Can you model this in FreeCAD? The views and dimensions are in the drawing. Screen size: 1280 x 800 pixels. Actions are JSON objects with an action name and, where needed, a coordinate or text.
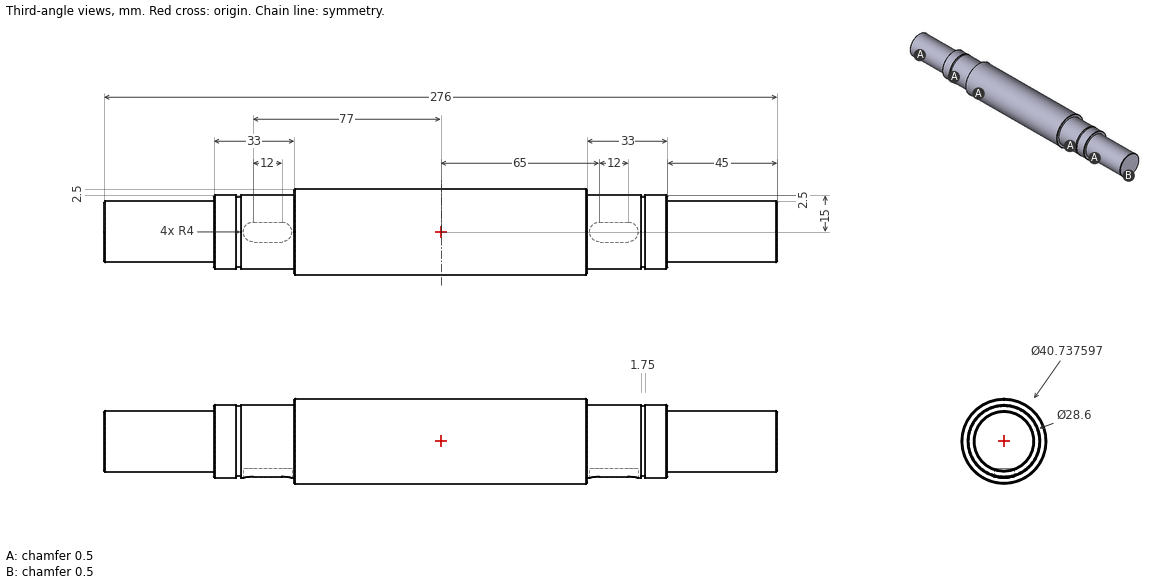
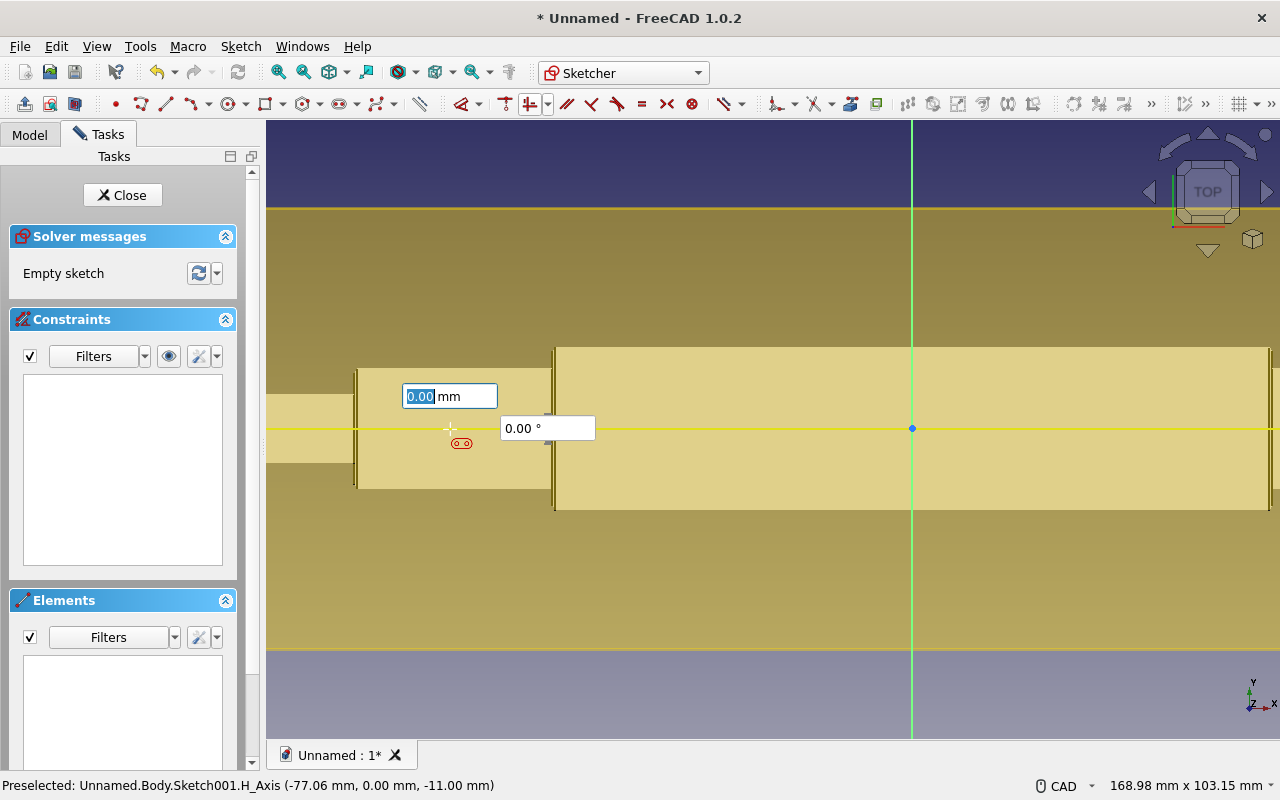
{"action": "left_click", "coordinate": [522, 420]}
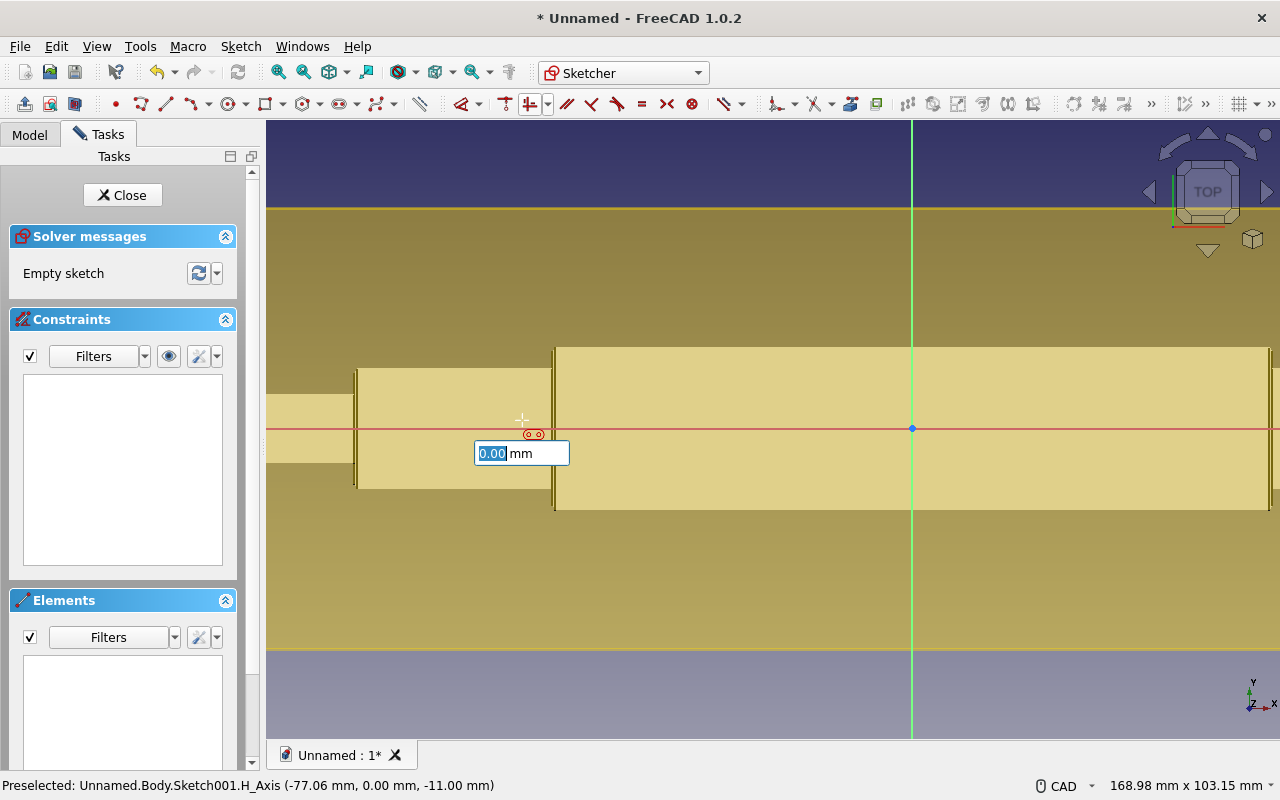
{"action": "left_click", "coordinate": [486, 405]}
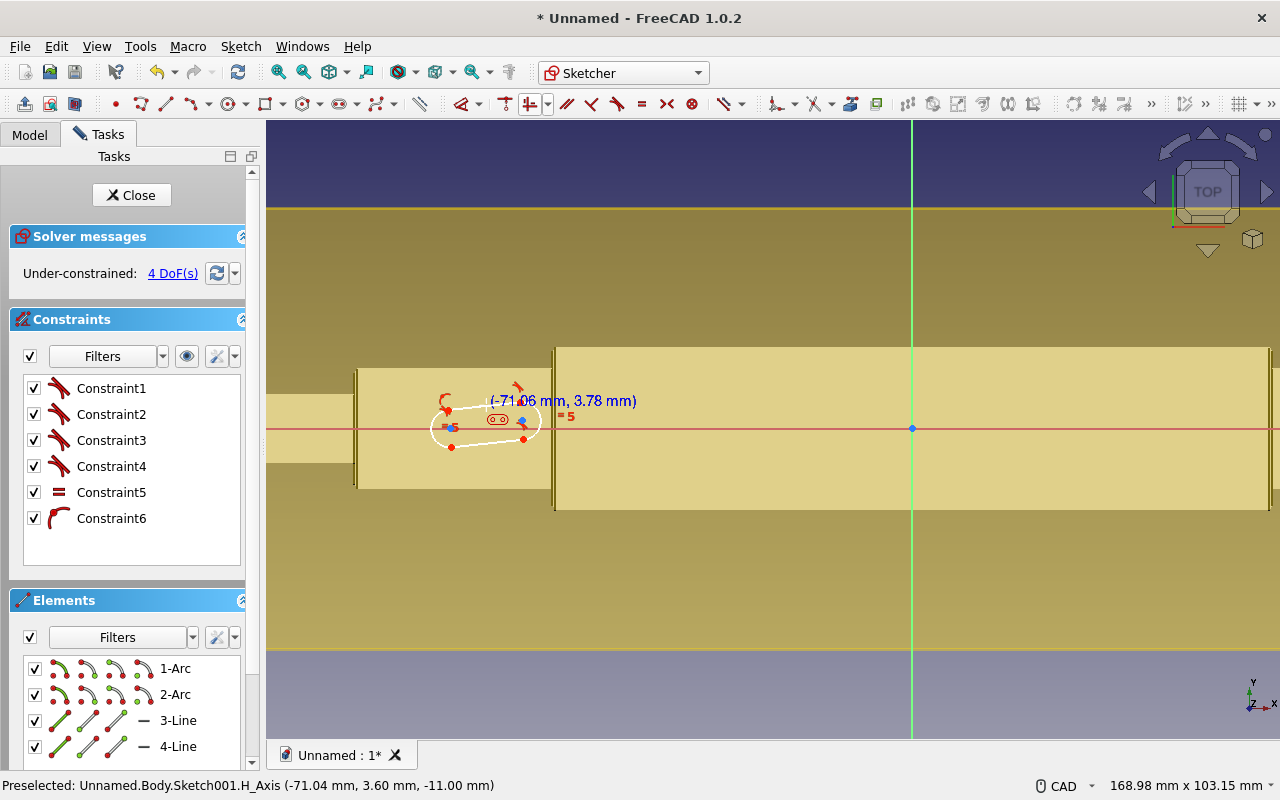
{"action": "scroll", "coordinate": [452, 431], "scroll_direction": "down", "scroll_amount": 3}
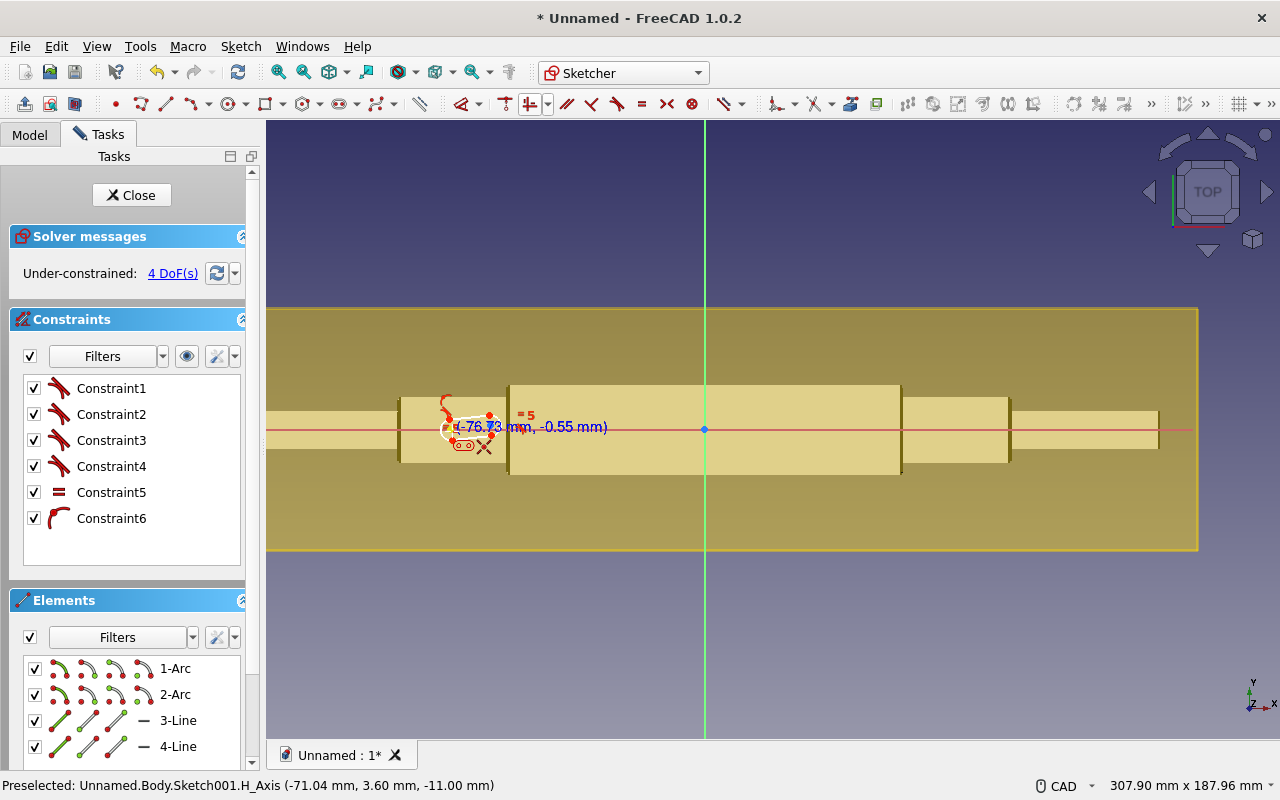
{"action": "scroll", "coordinate": [919, 430], "scroll_direction": "up", "scroll_amount": 3}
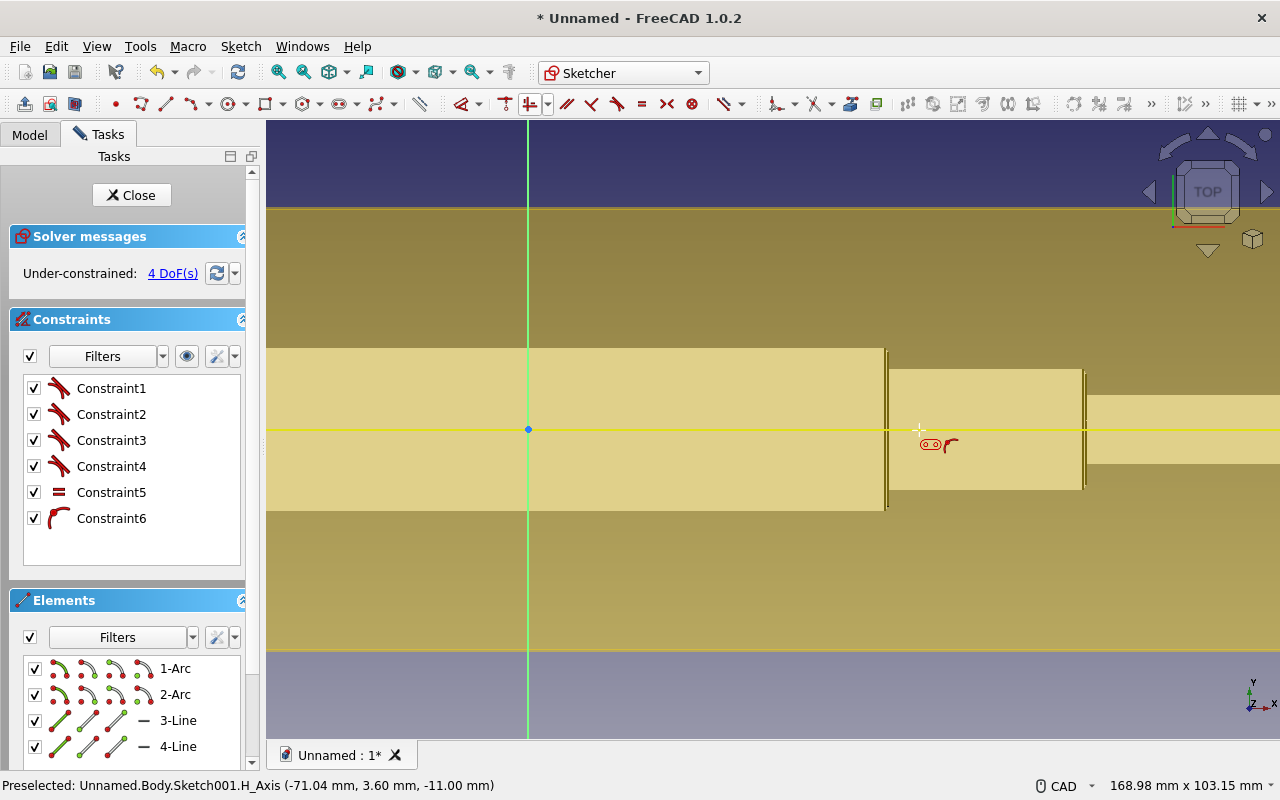
{"action": "left_click", "coordinate": [918, 430]}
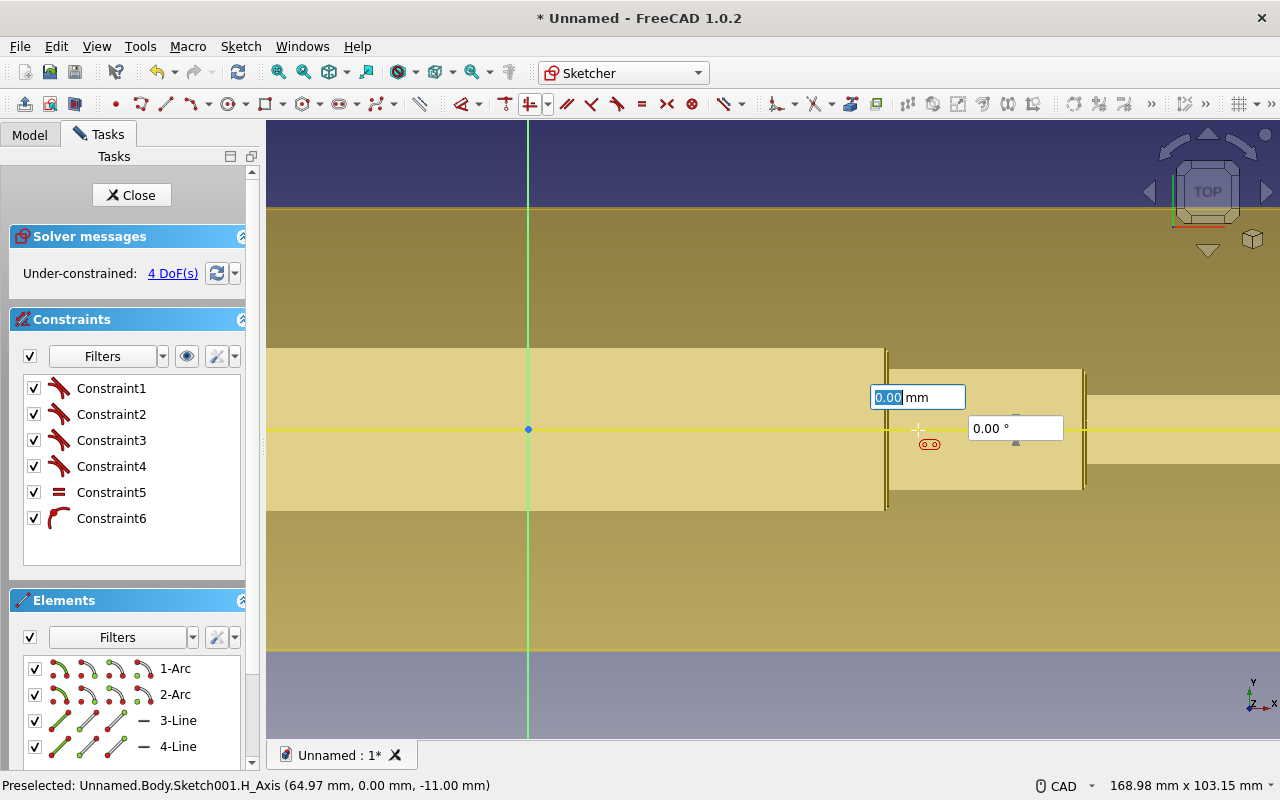
{"action": "left_click", "coordinate": [990, 421]}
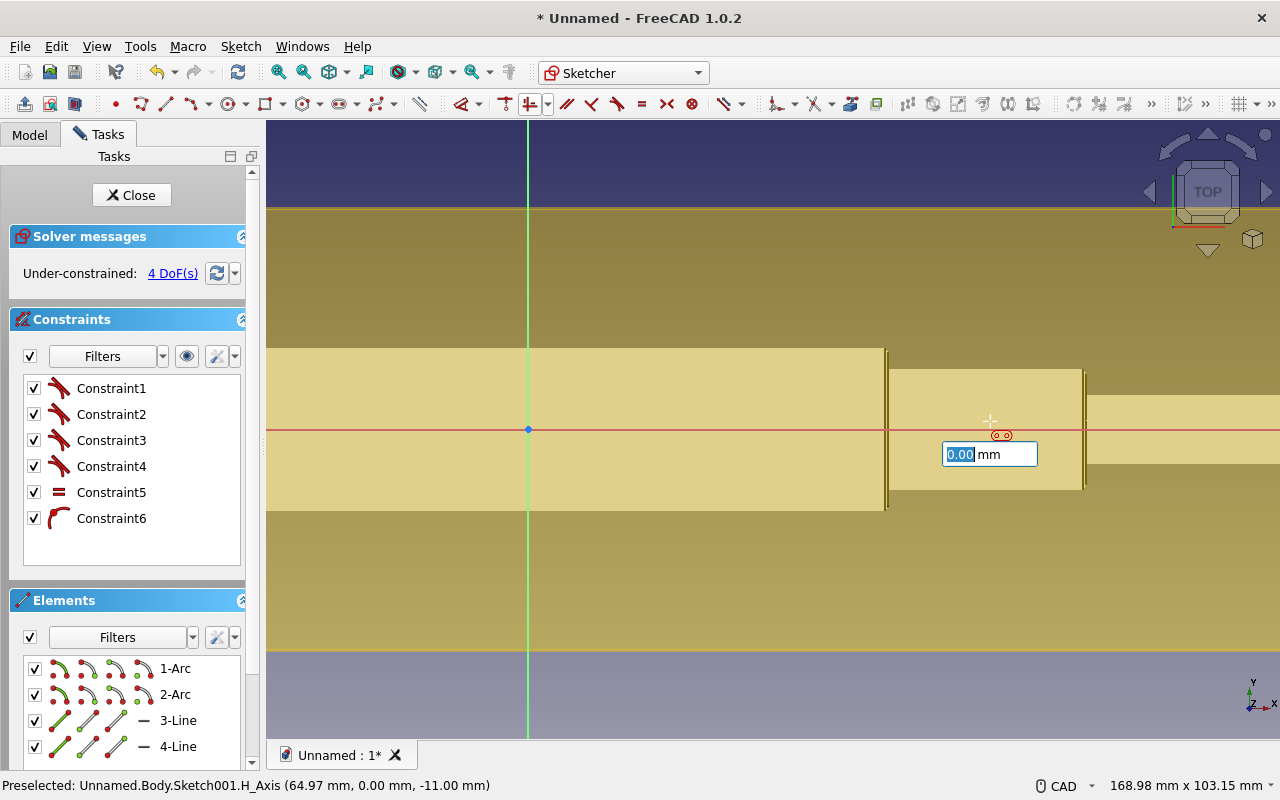
{"action": "left_click", "coordinate": [954, 405]}
{"action": "key", "text": "Escape"}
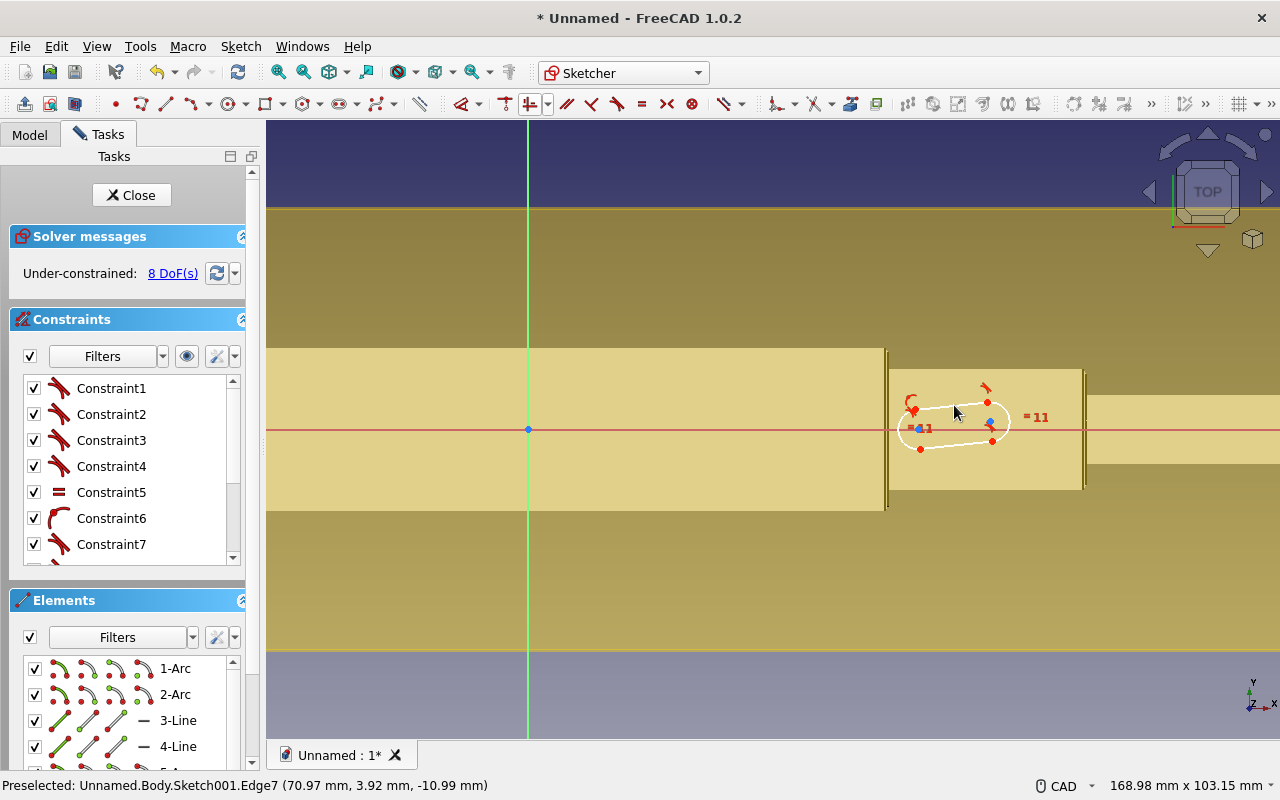
{"action": "scroll", "coordinate": [919, 429], "scroll_direction": "down", "scroll_amount": 3}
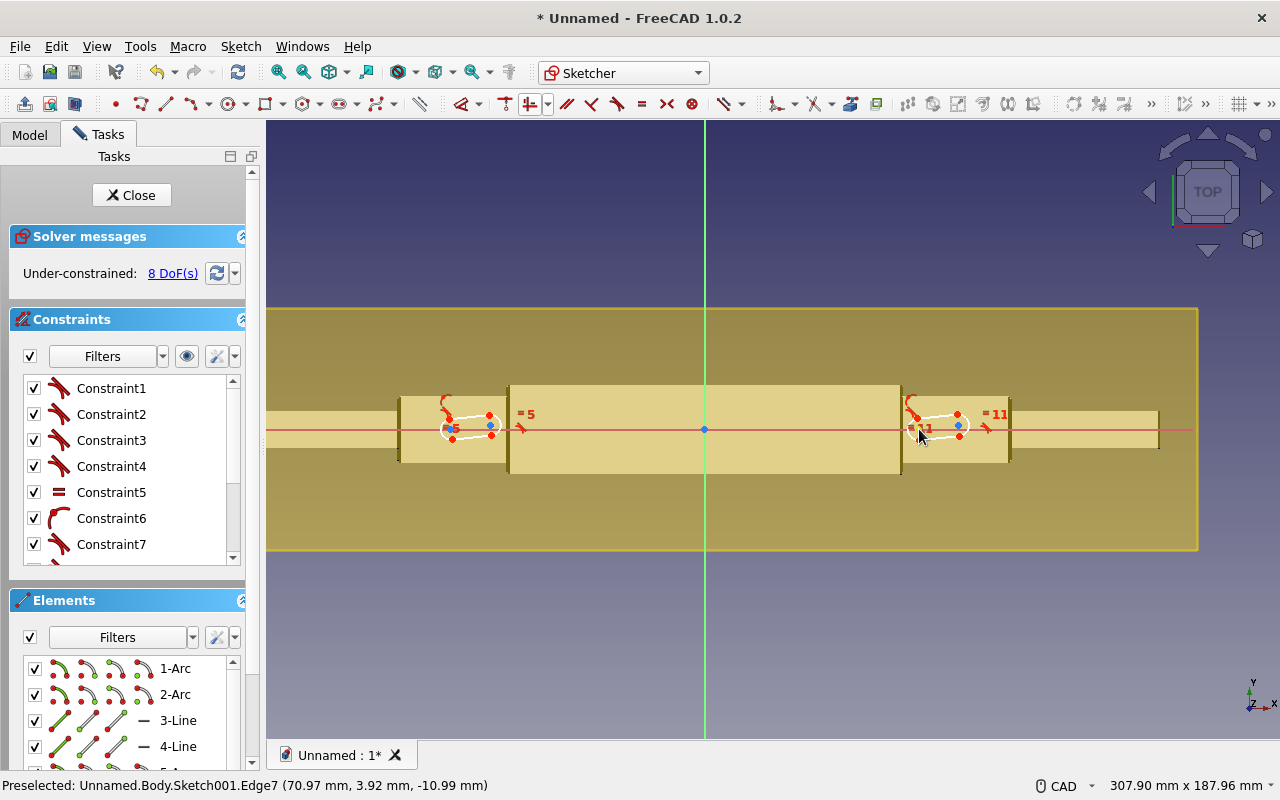
{"action": "left_click", "coordinate": [462, 418]}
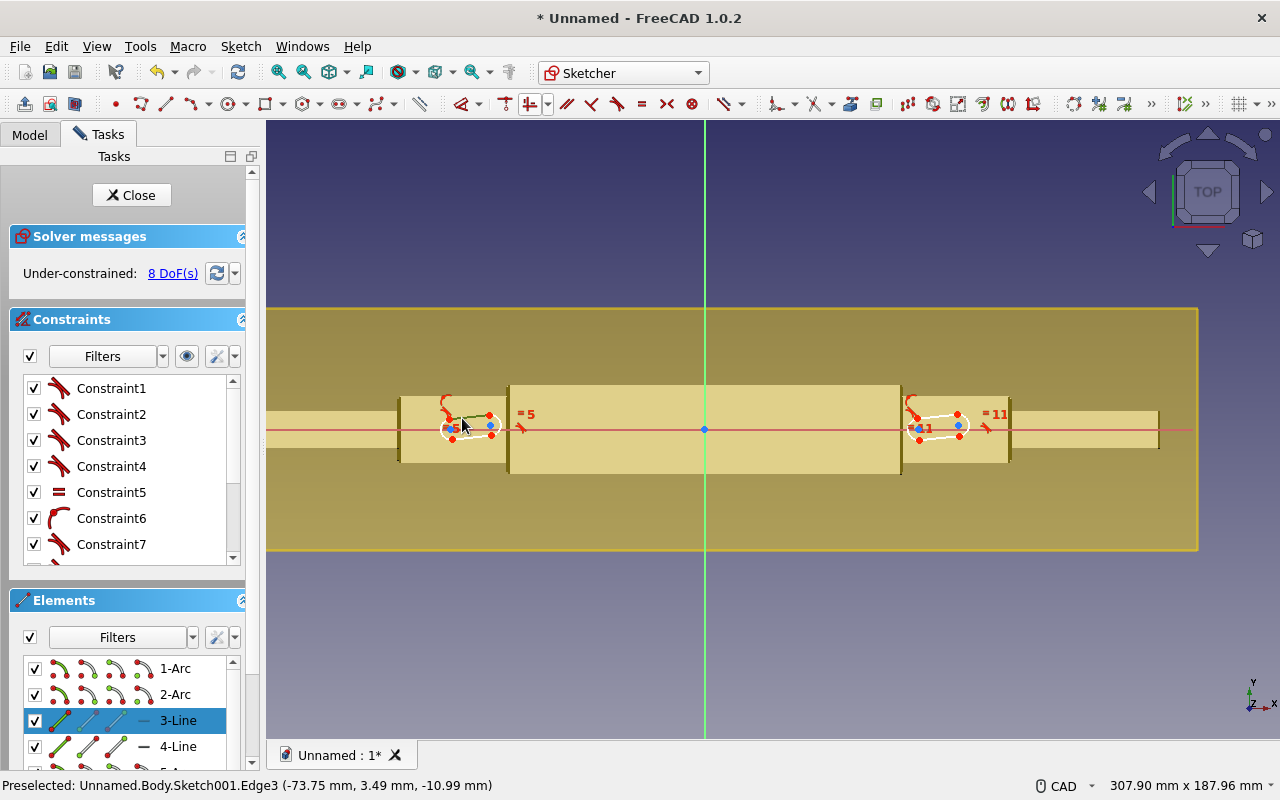
{"action": "left_click", "coordinate": [548, 104]}